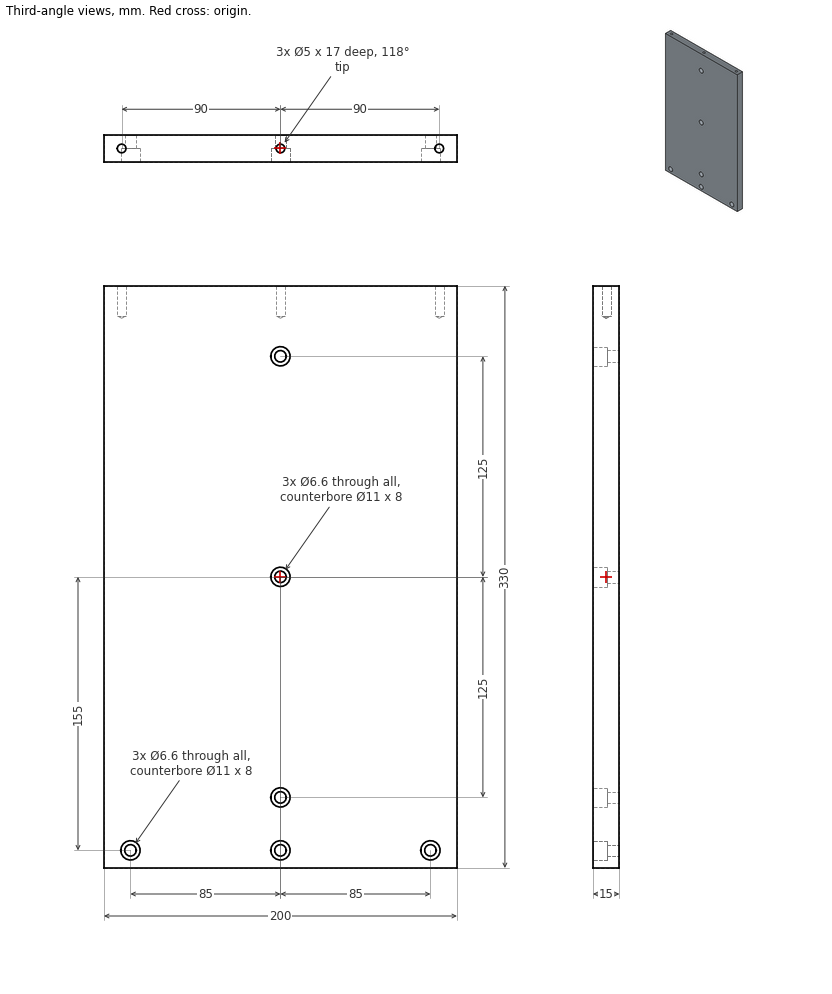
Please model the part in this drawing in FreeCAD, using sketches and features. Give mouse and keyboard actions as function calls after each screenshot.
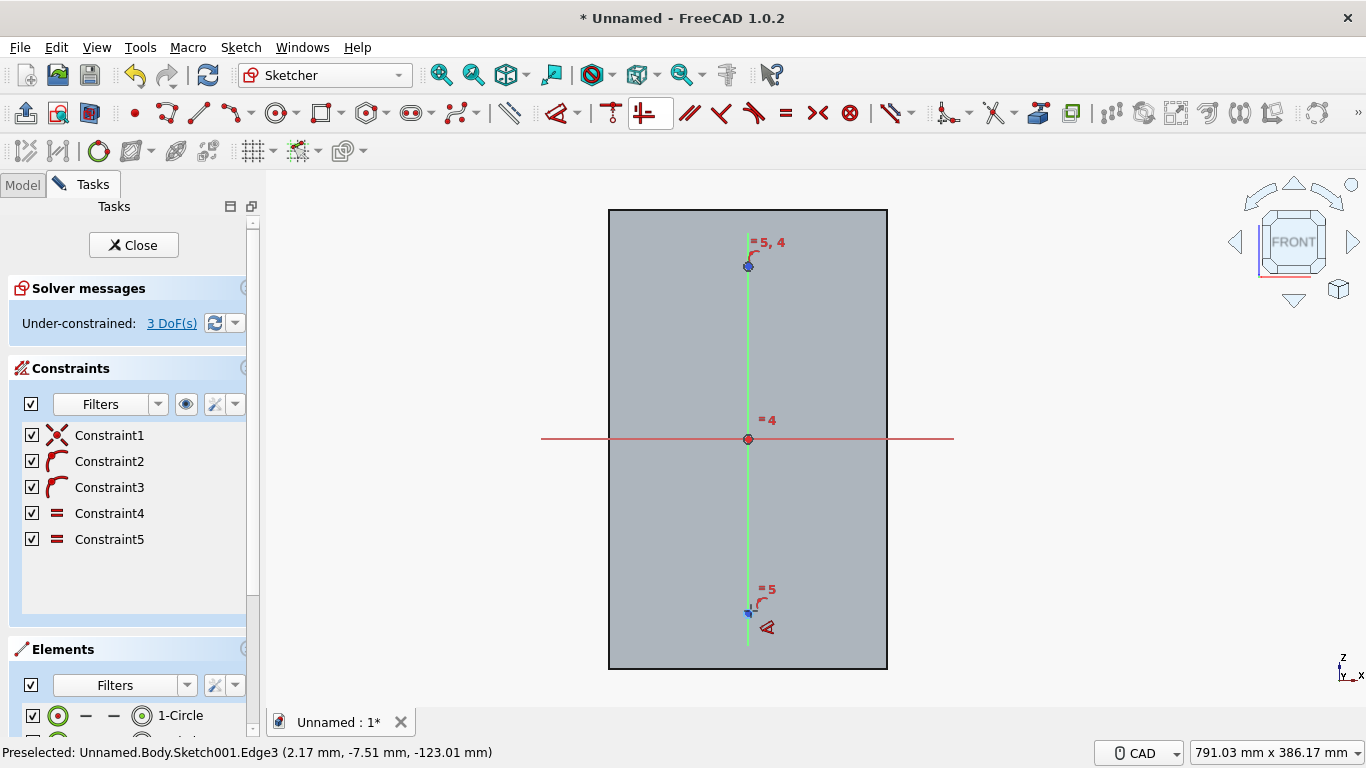
scroll(751, 436, up, 8)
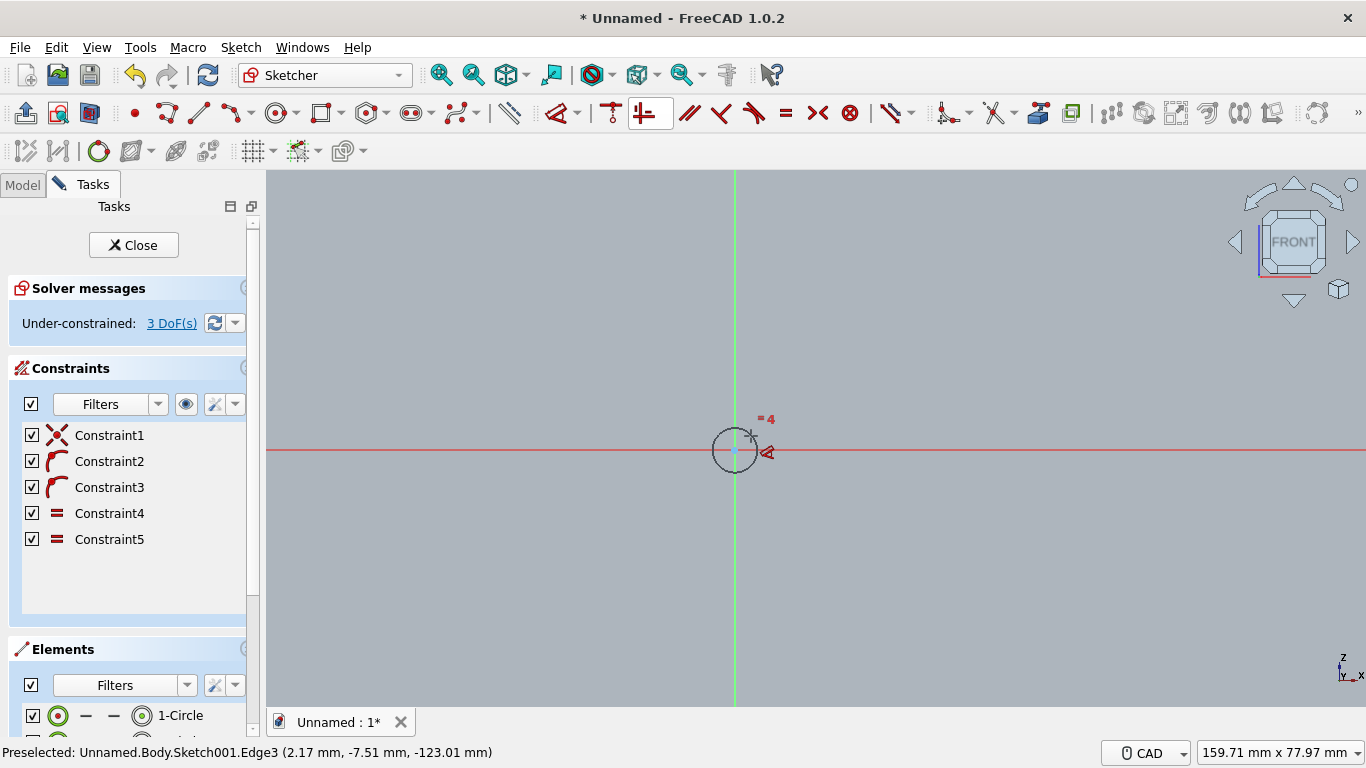
click(751, 435)
click(774, 413)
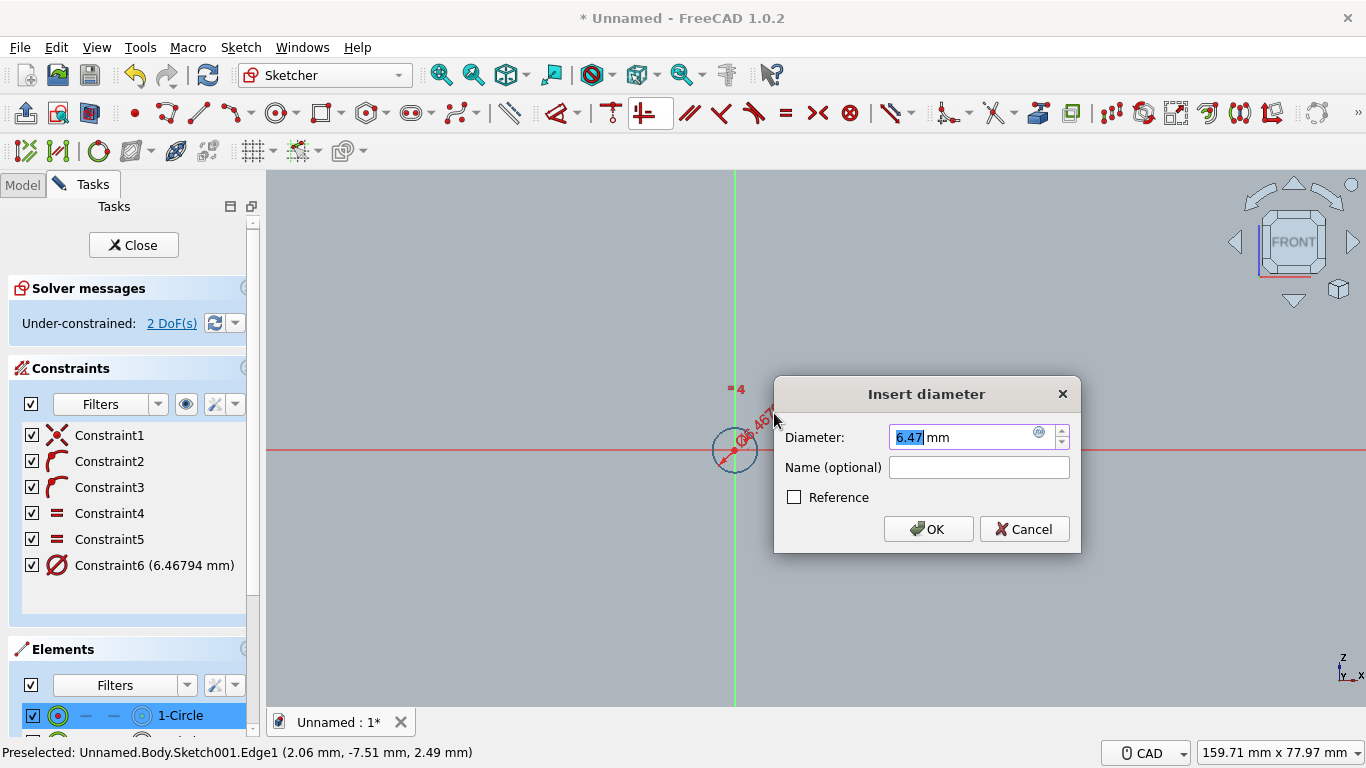
text(6.6)
key(Return)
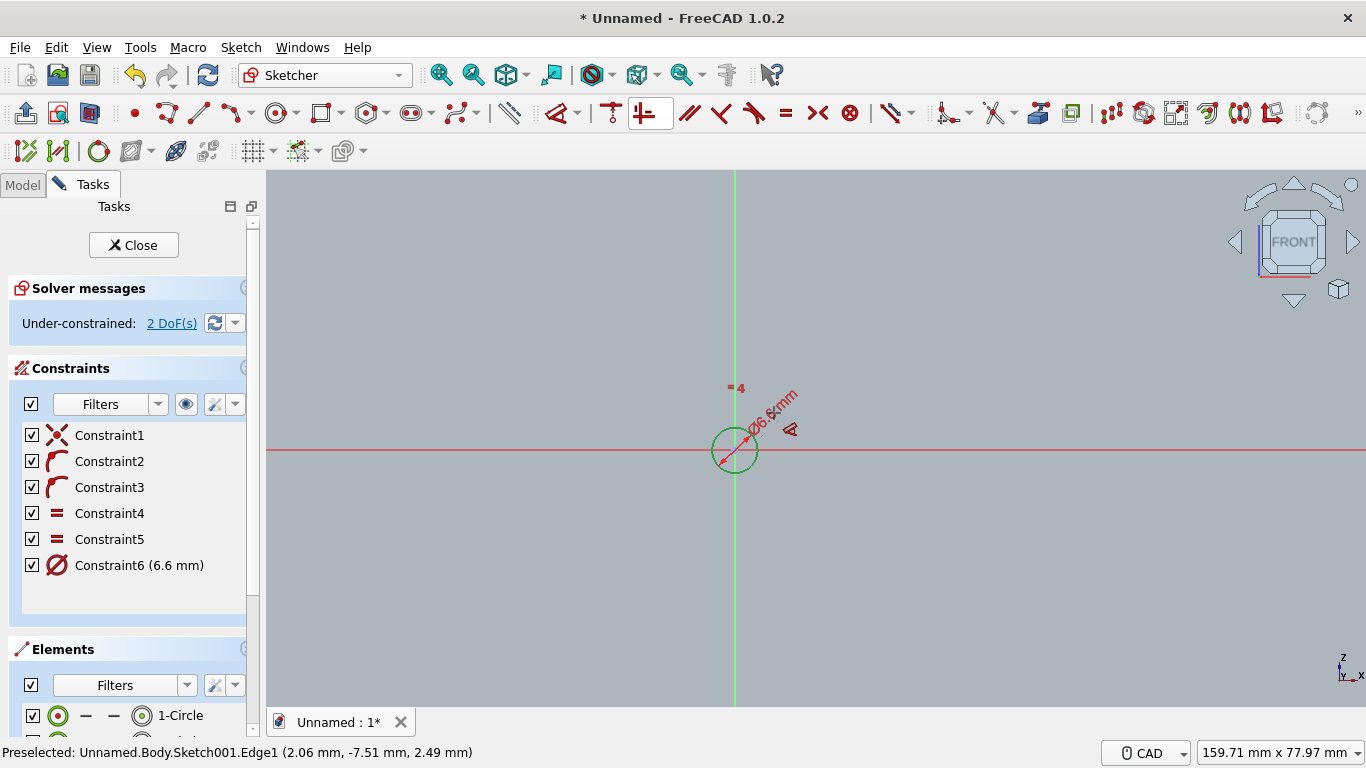
scroll(751, 435, down, 8)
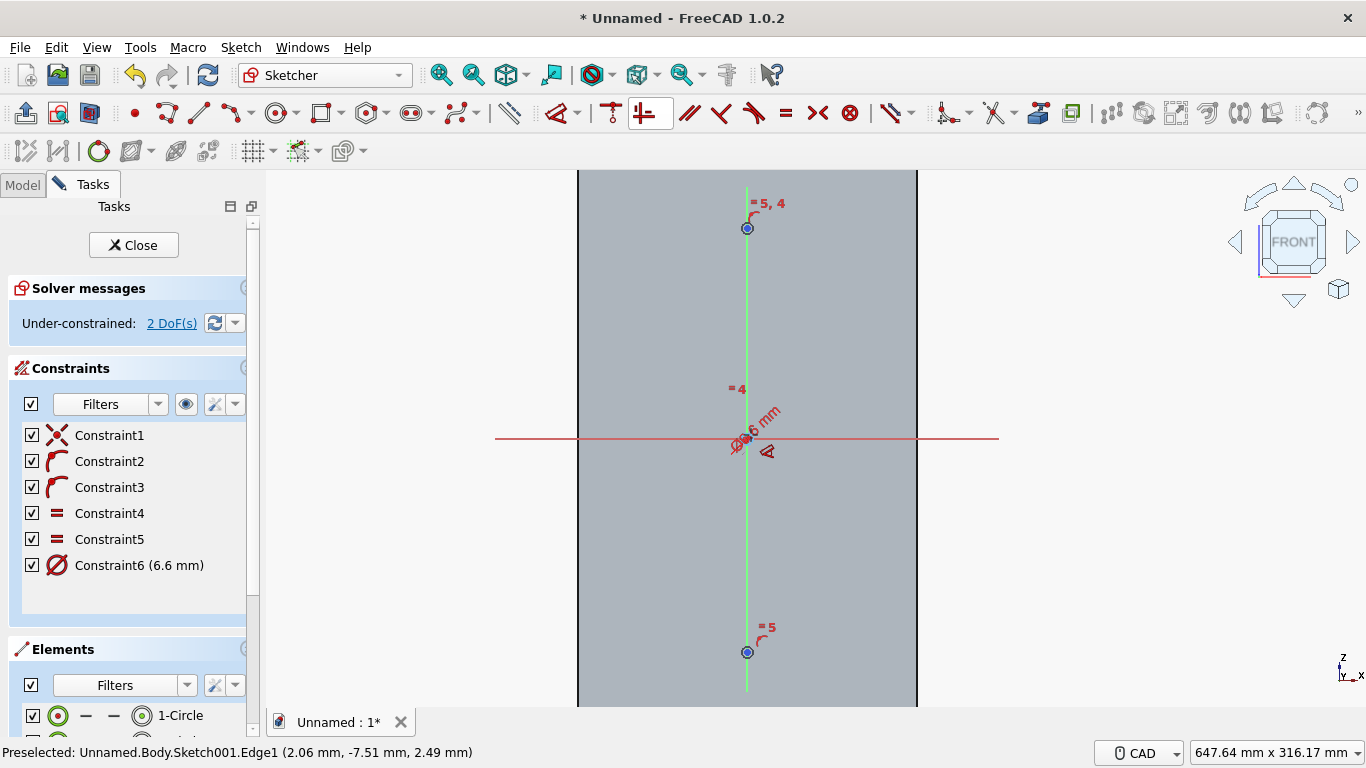
click(748, 266)
click(782, 352)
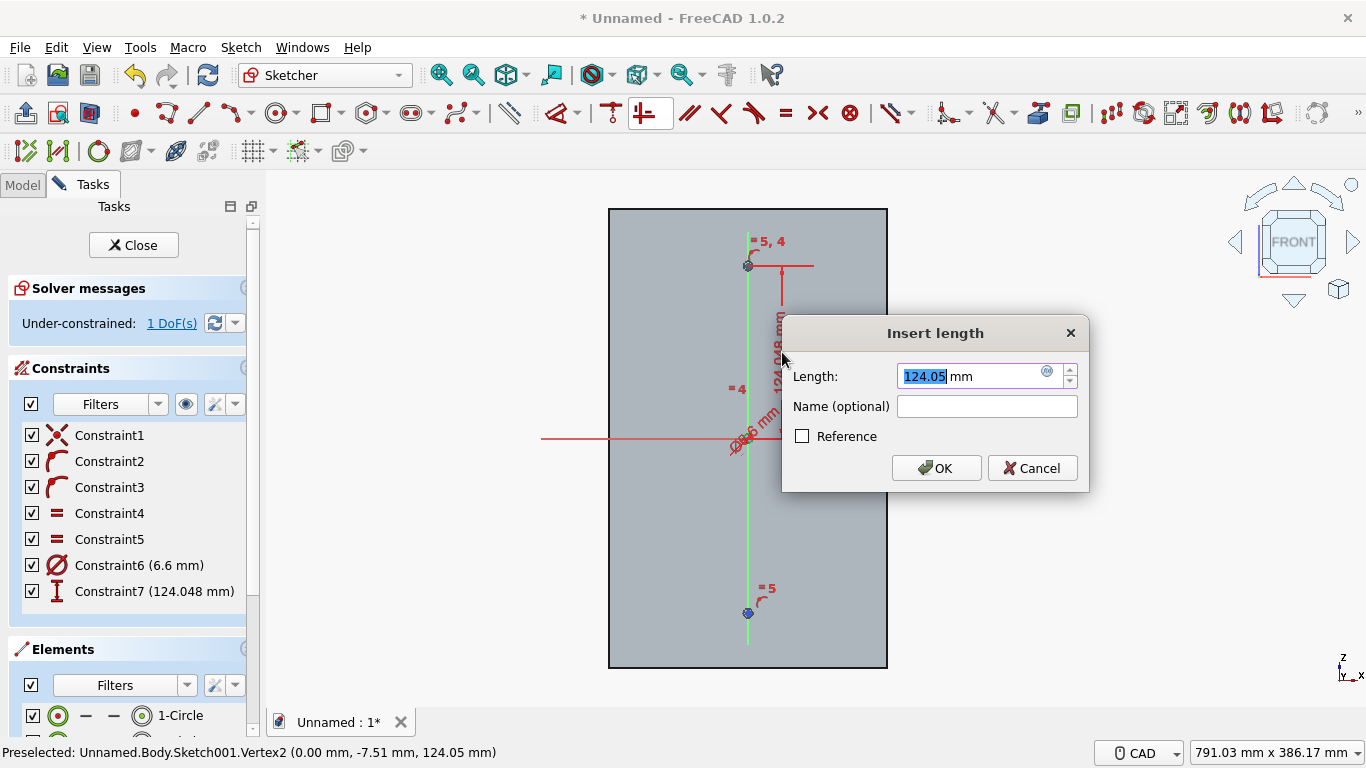
text(125)
key(Return)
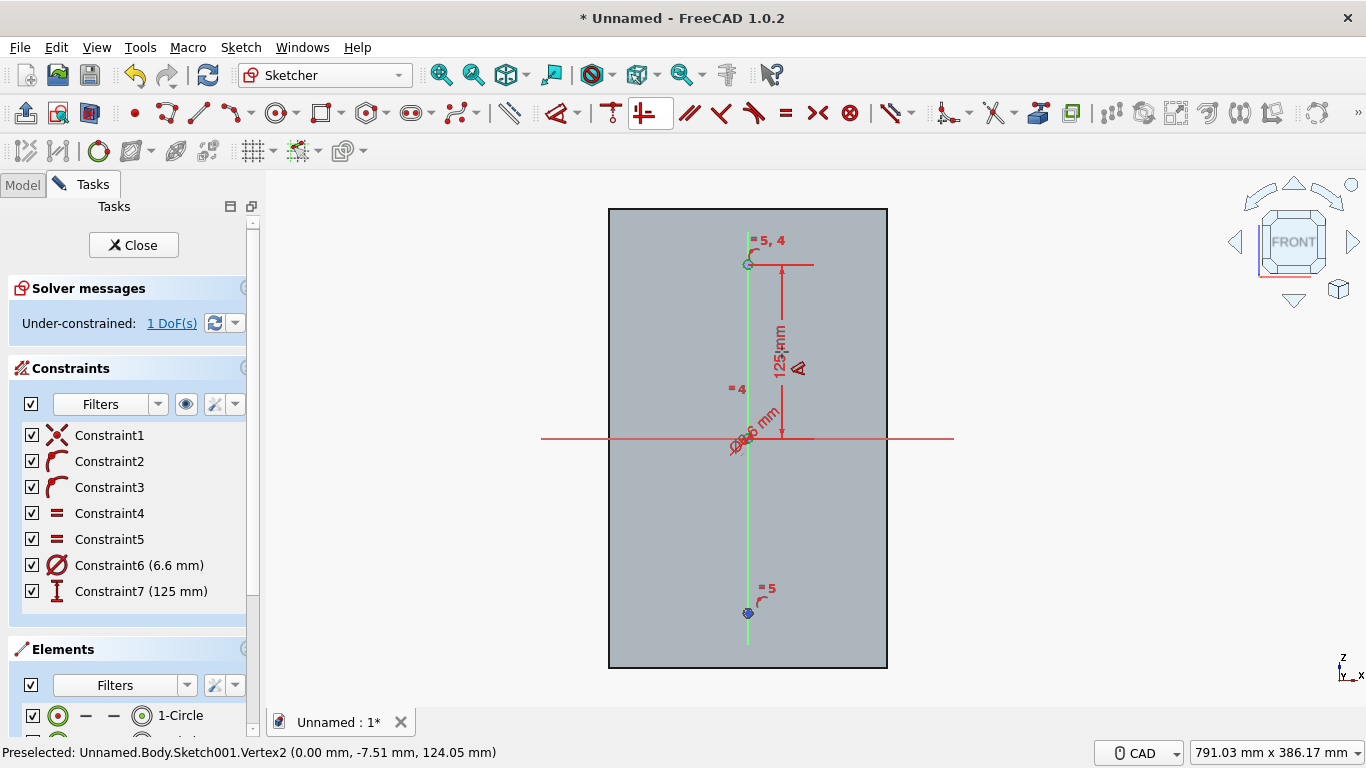
click(748, 613)
click(782, 526)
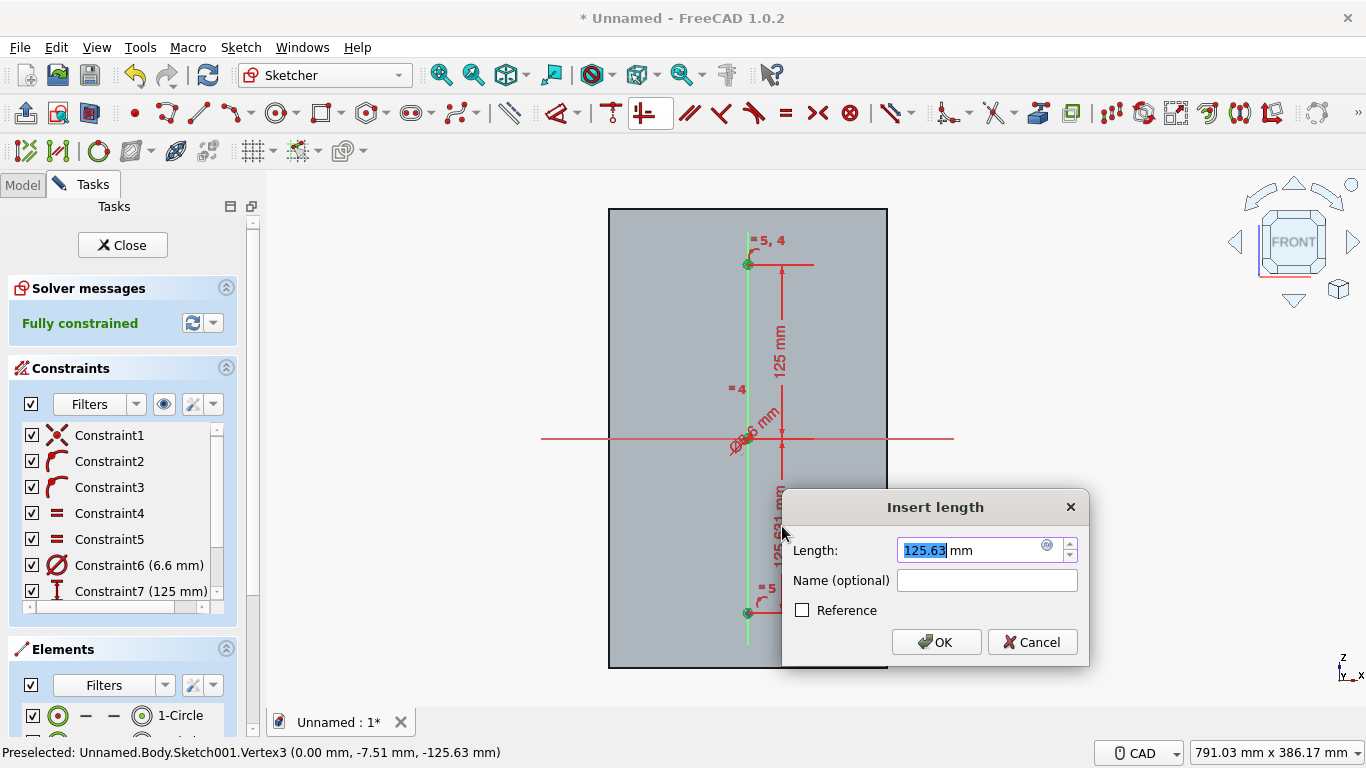
text(125)
key(Return)
key(Escape)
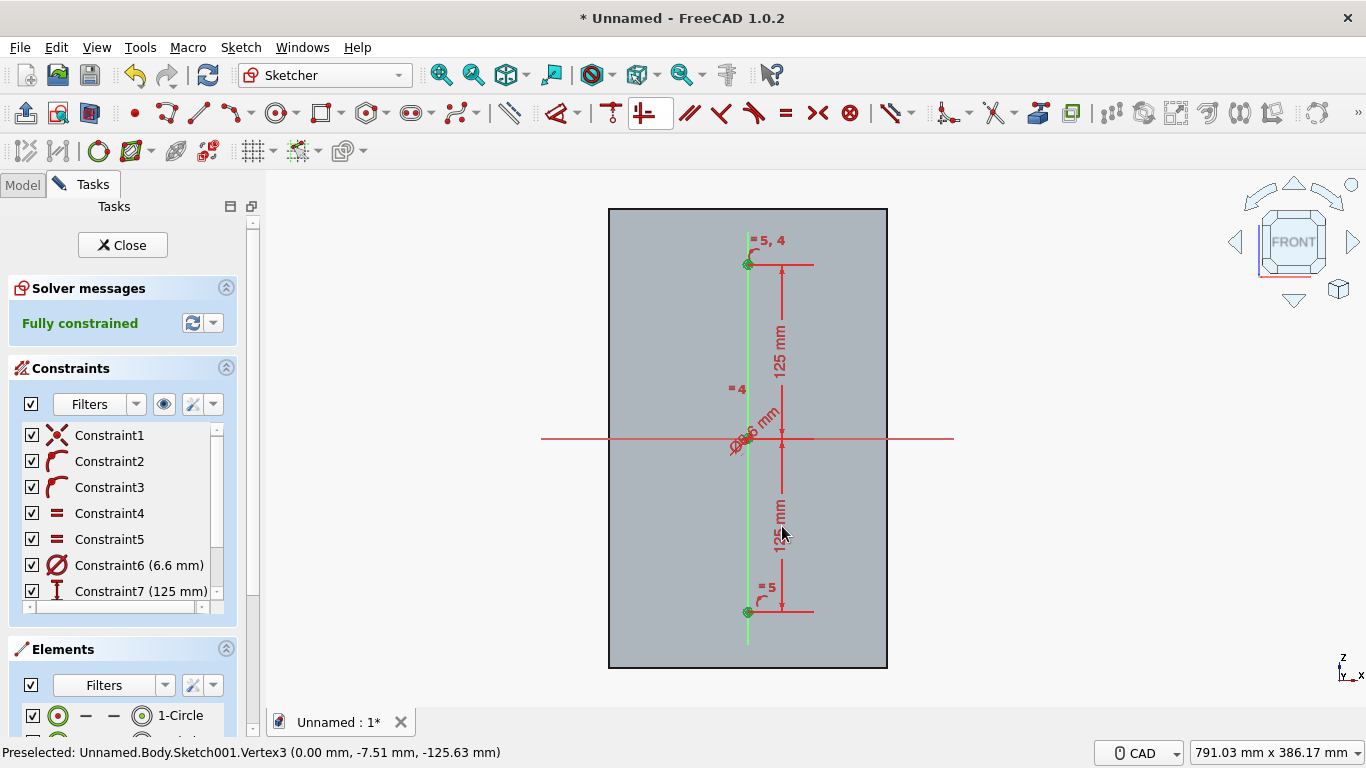
click(123, 245)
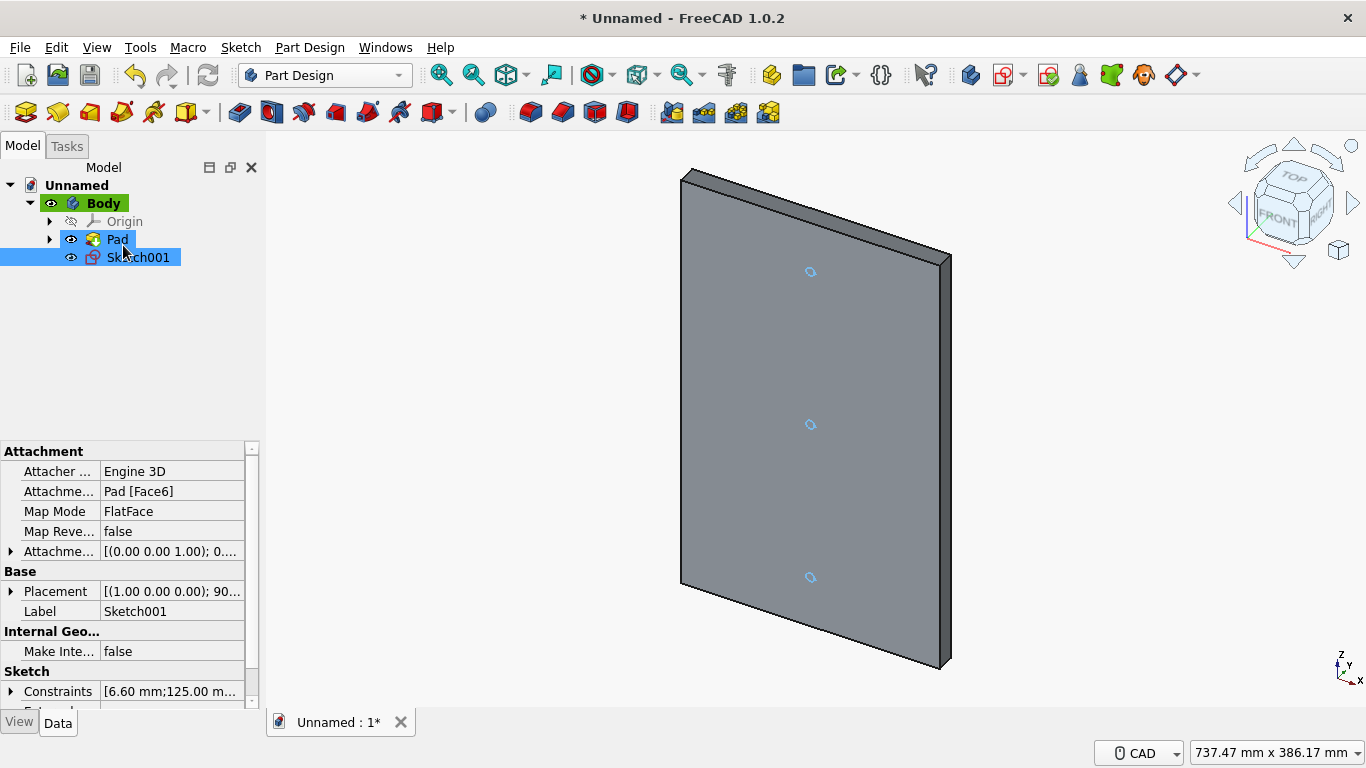
click(272, 112)